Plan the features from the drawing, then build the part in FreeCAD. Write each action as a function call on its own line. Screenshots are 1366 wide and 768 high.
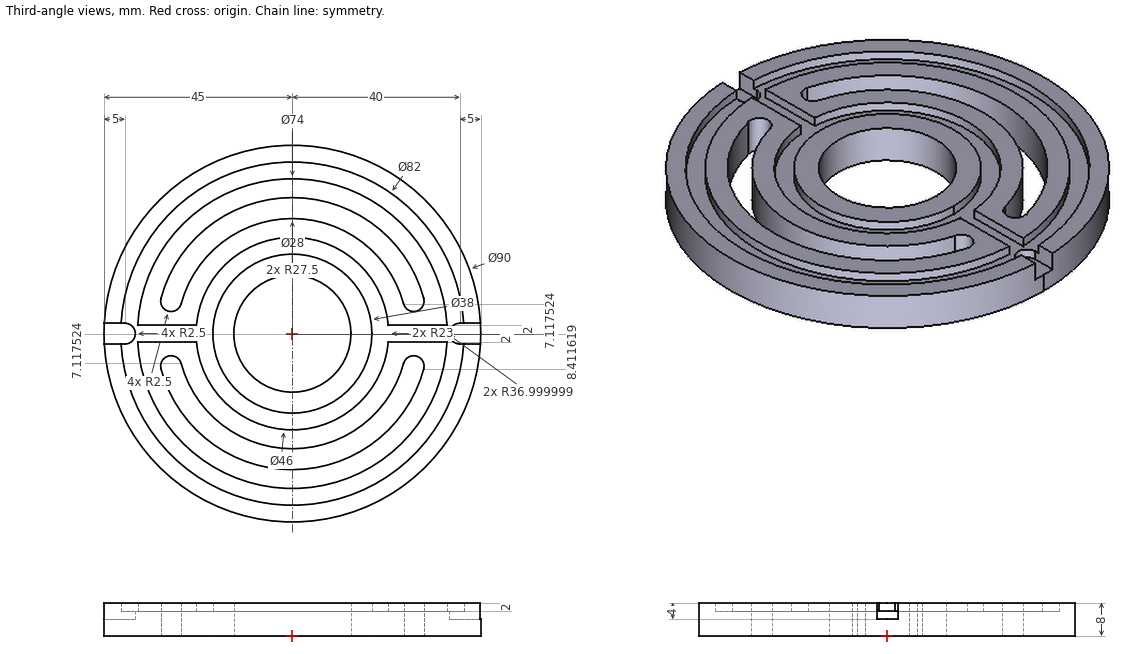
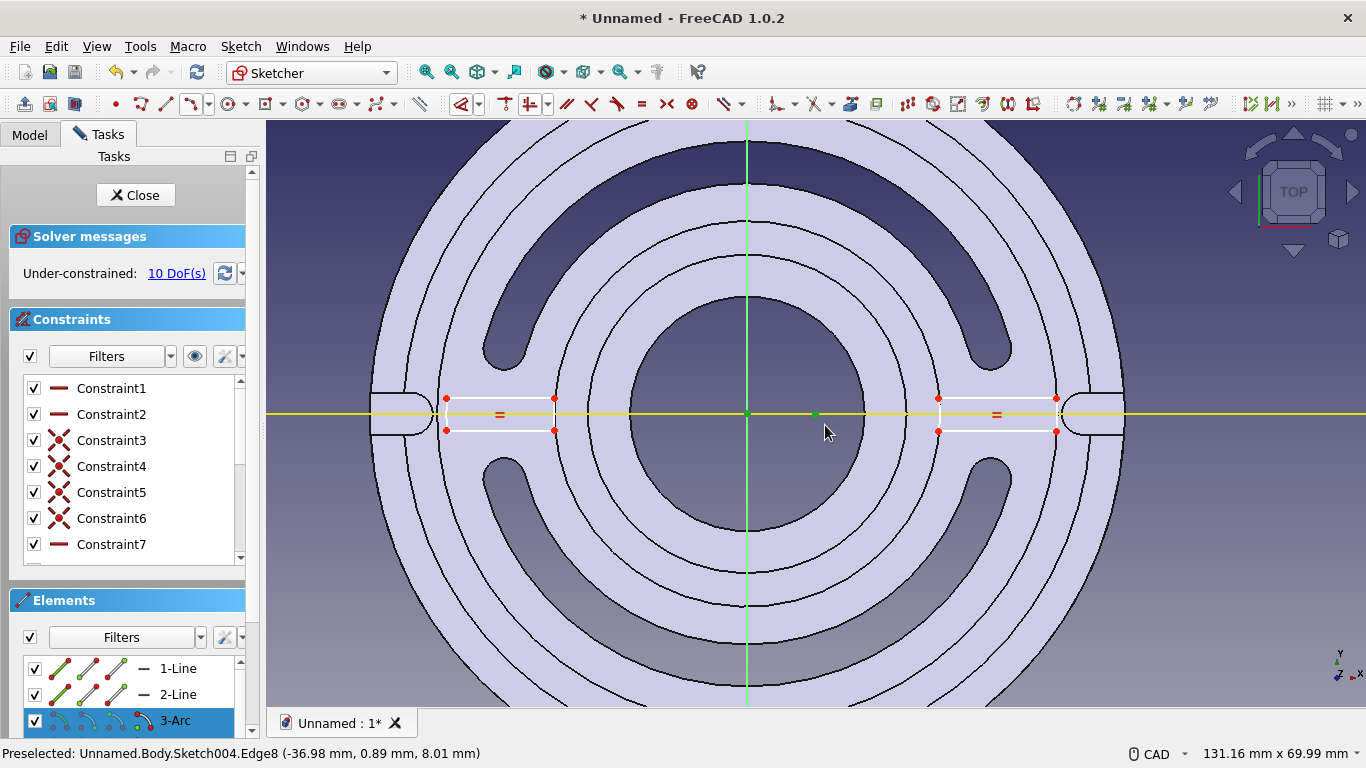
key(c)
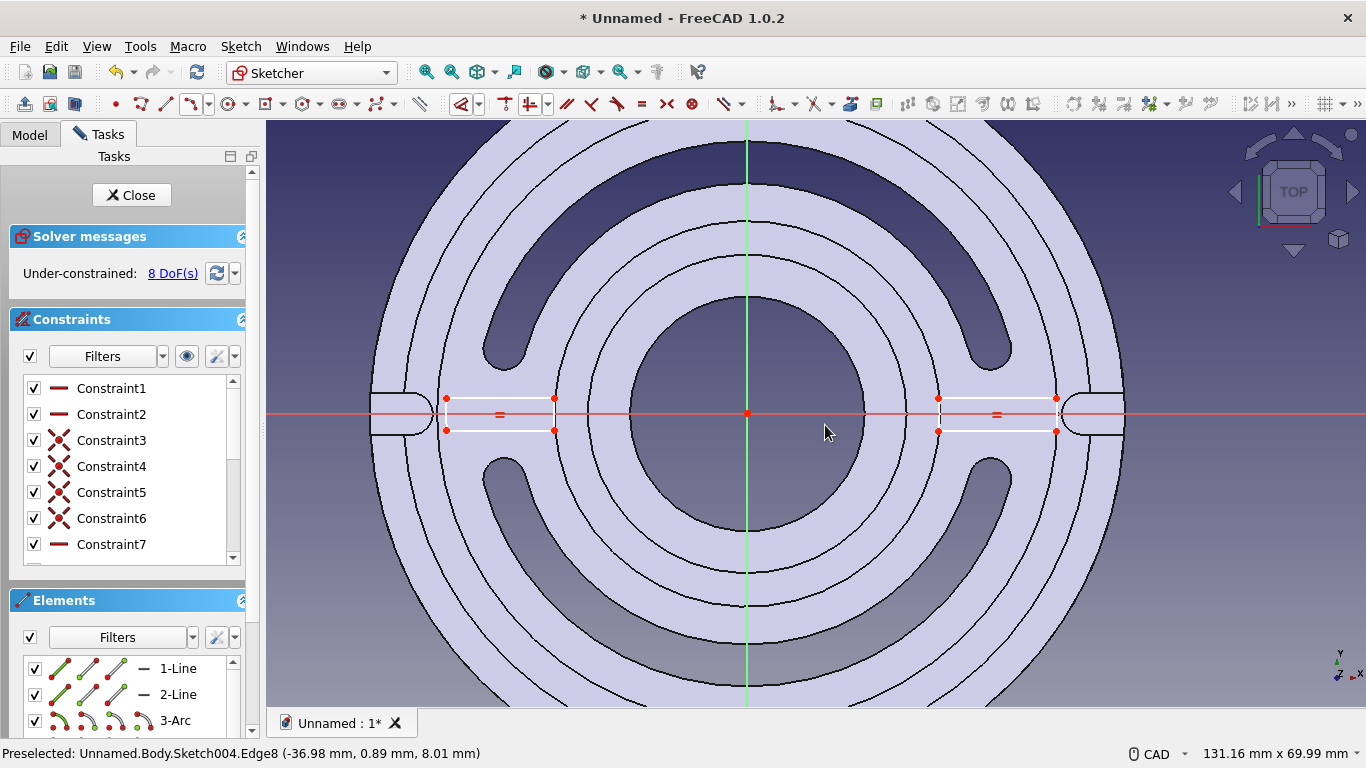
click(1057, 431)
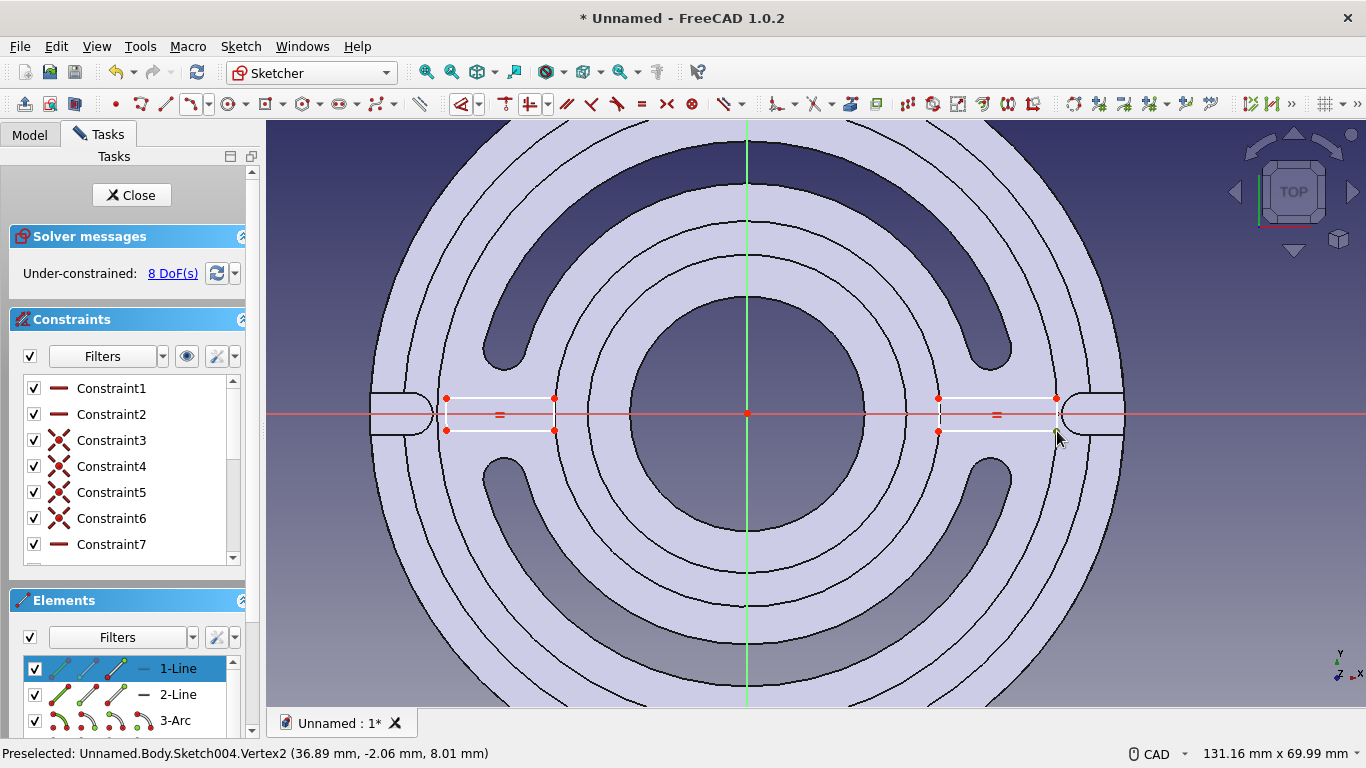
click(447, 431)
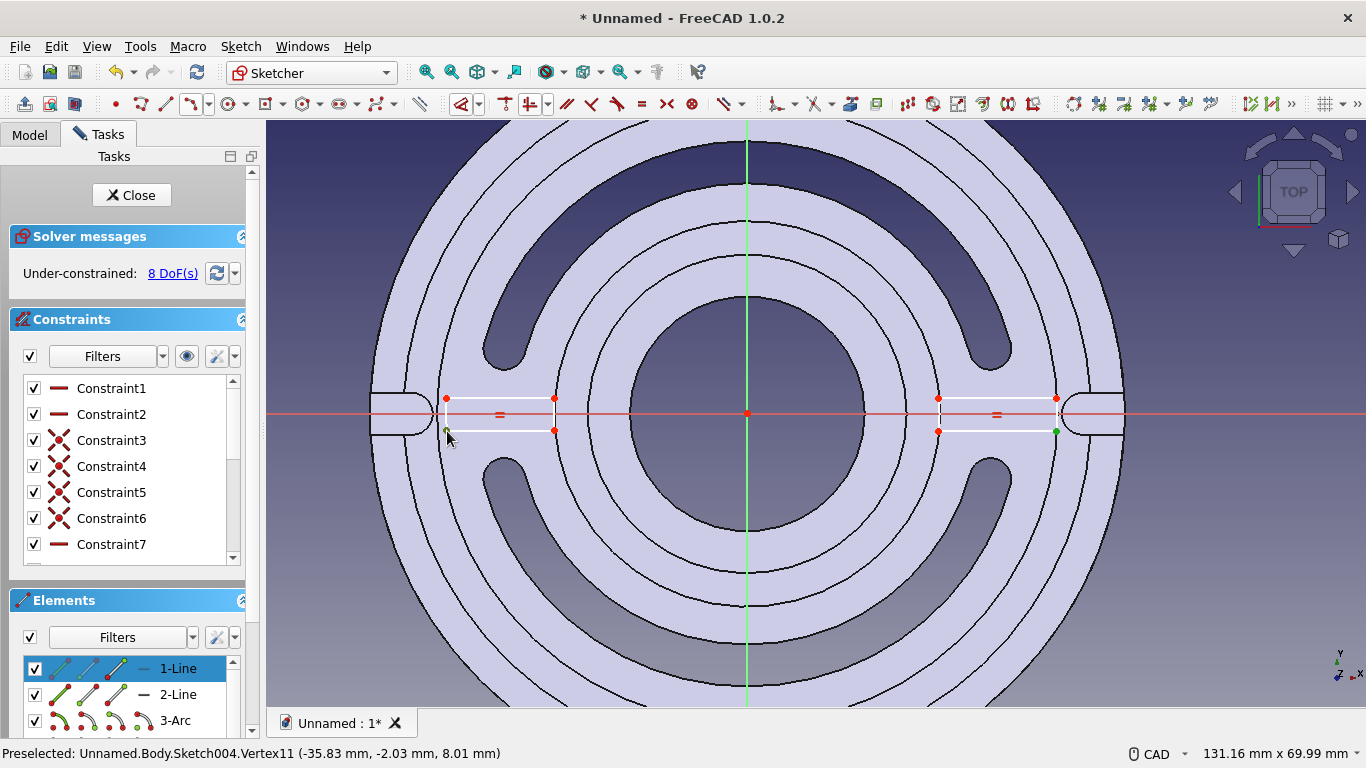
click(747, 641)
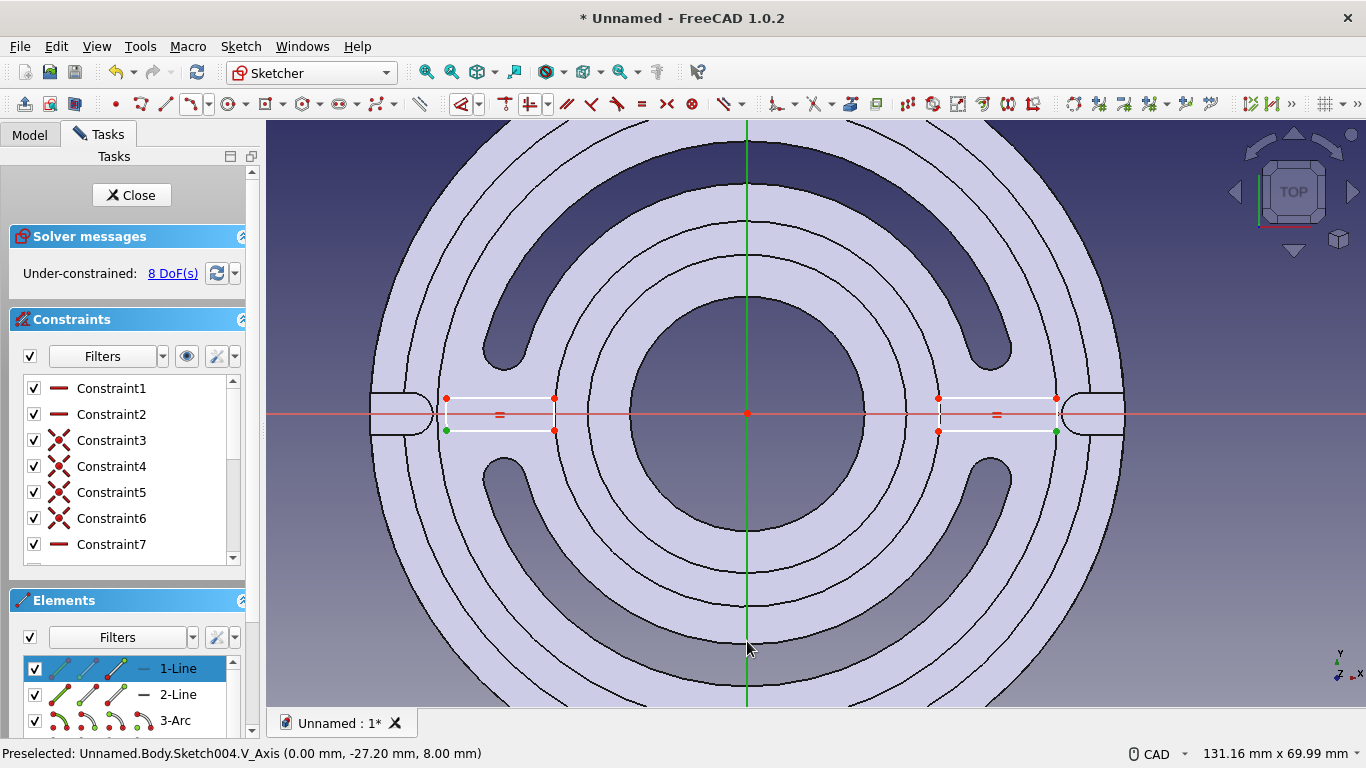
click(667, 104)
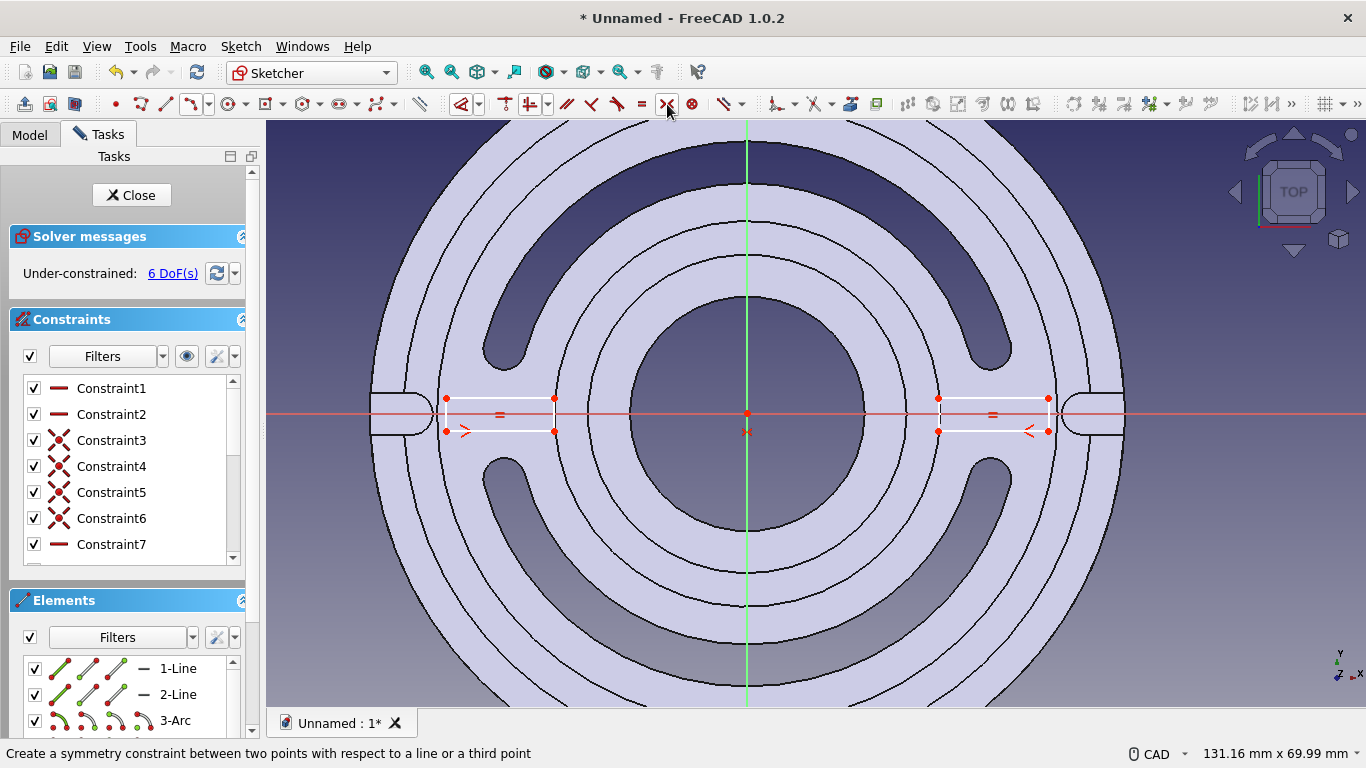
click(939, 398)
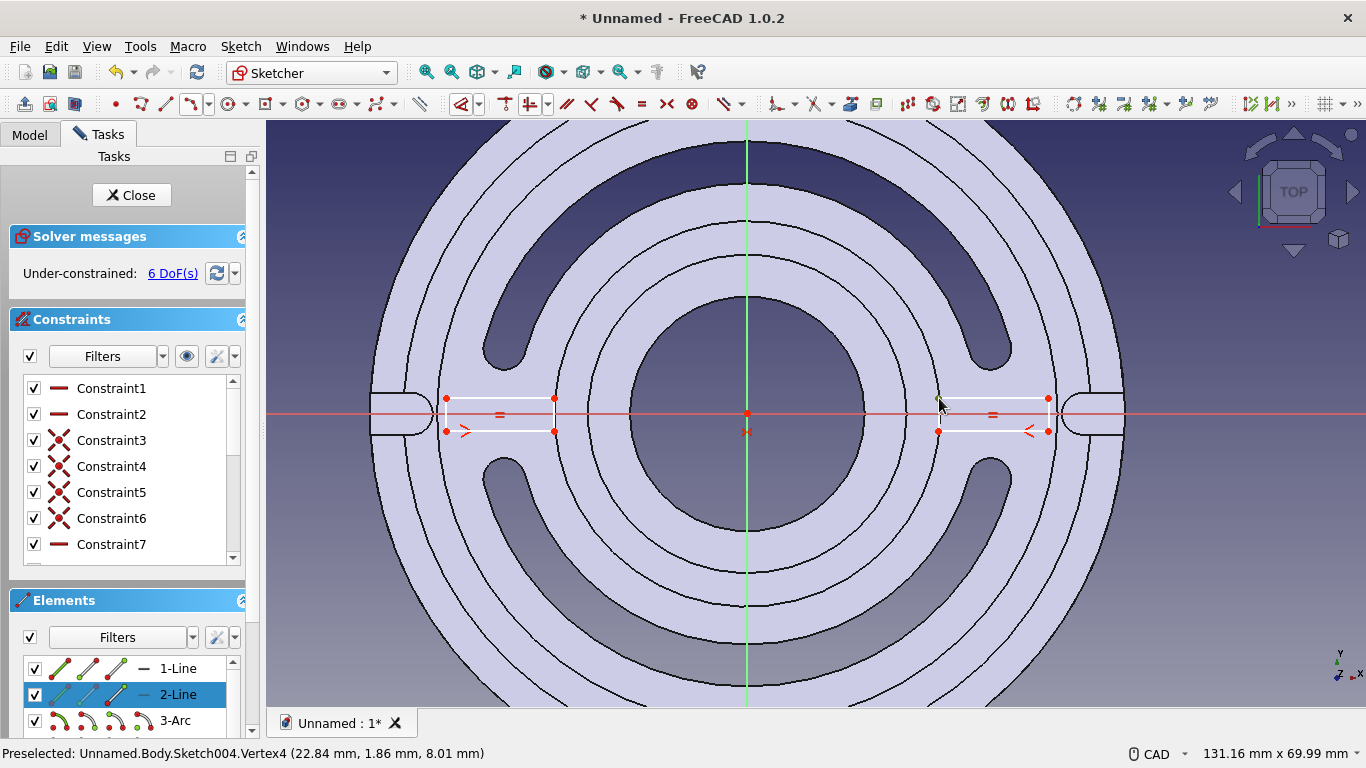
click(555, 398)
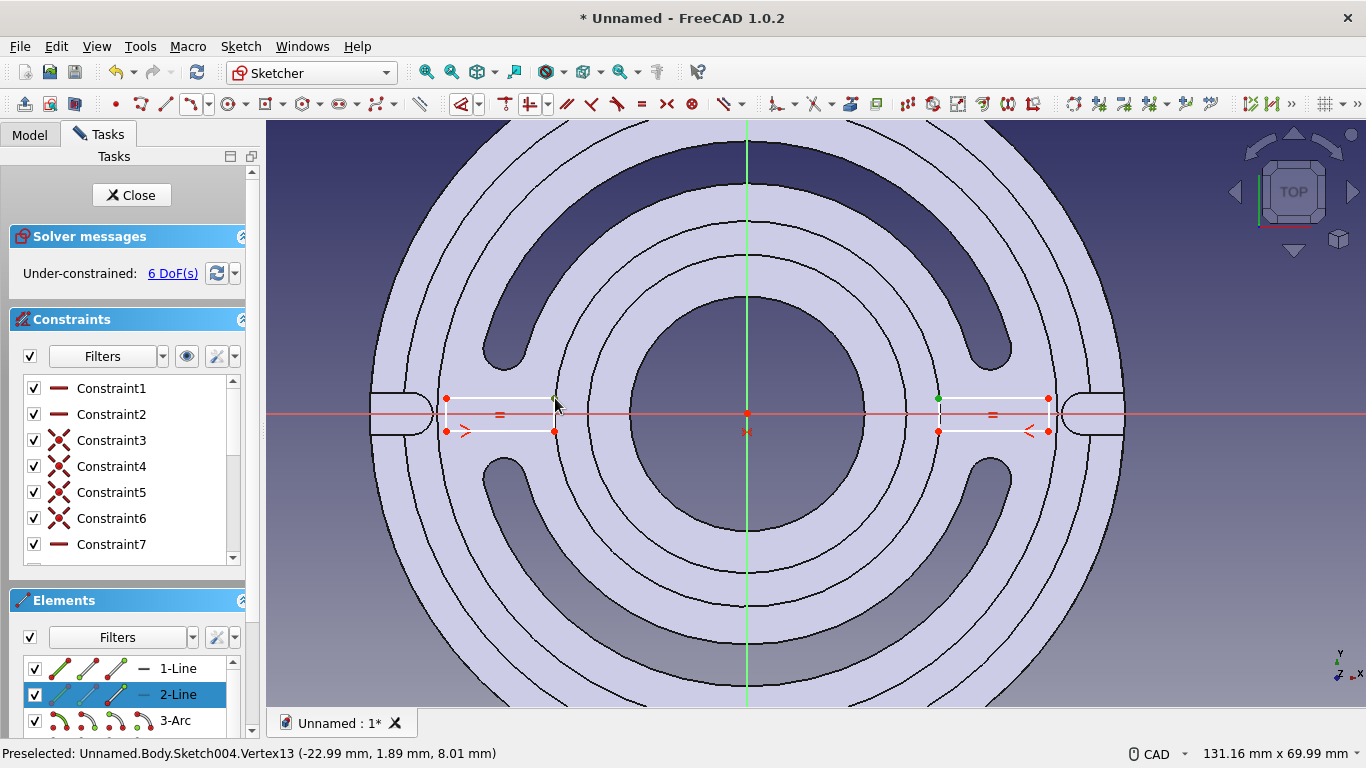
click(747, 641)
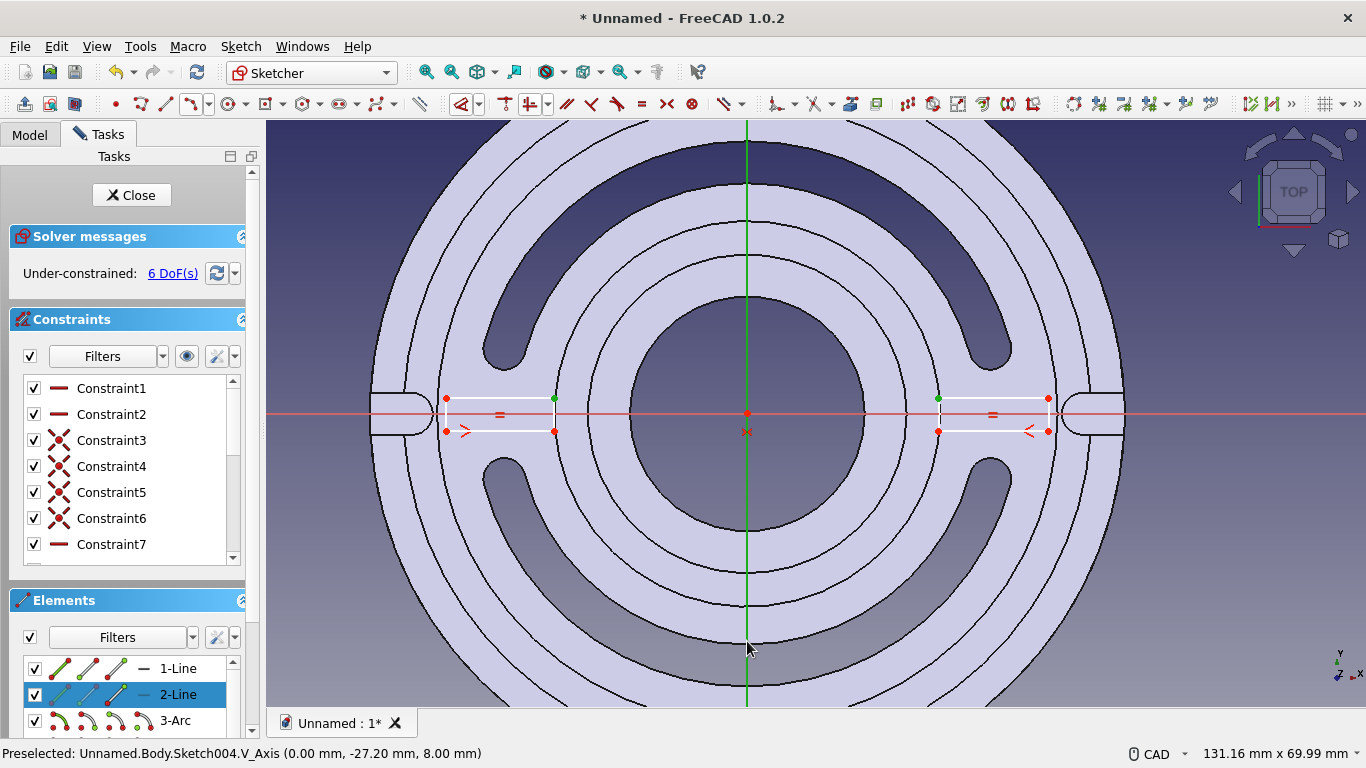
key(s)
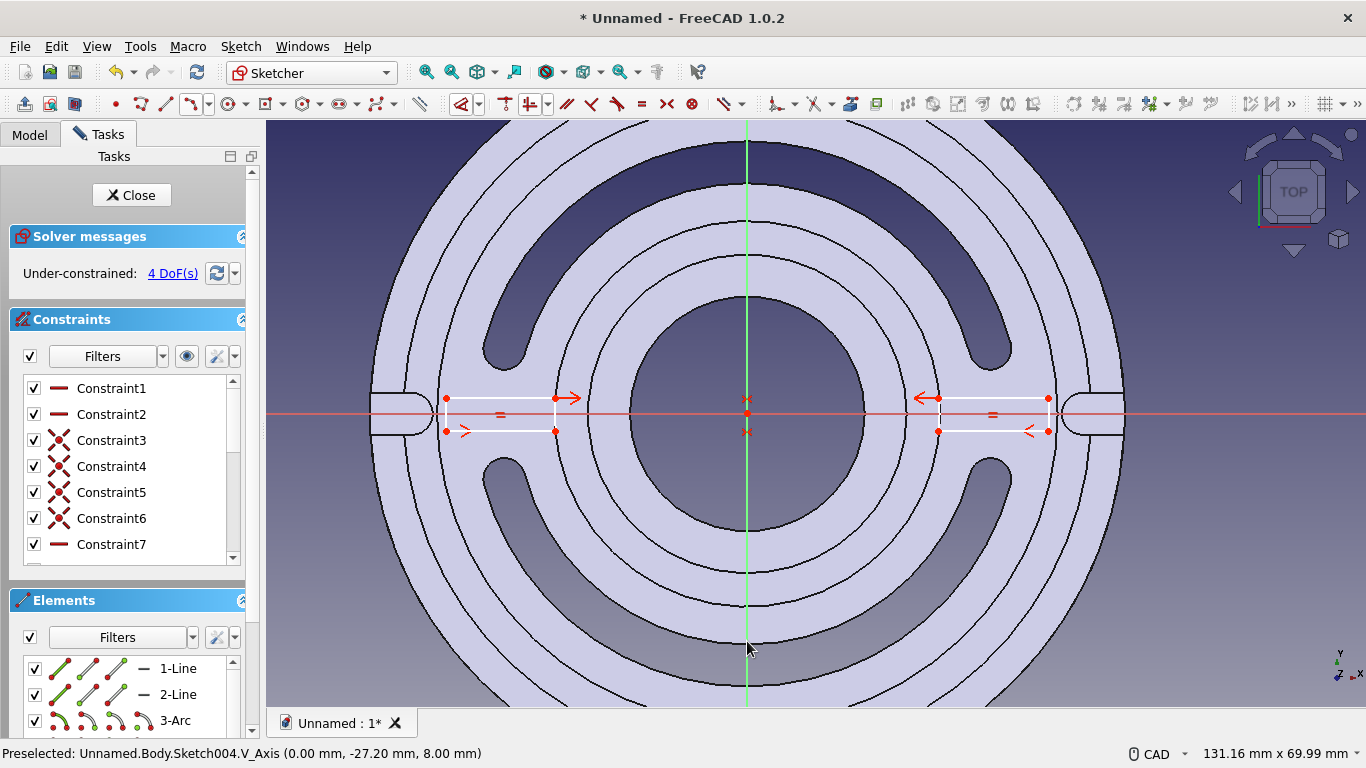
click(460, 104)